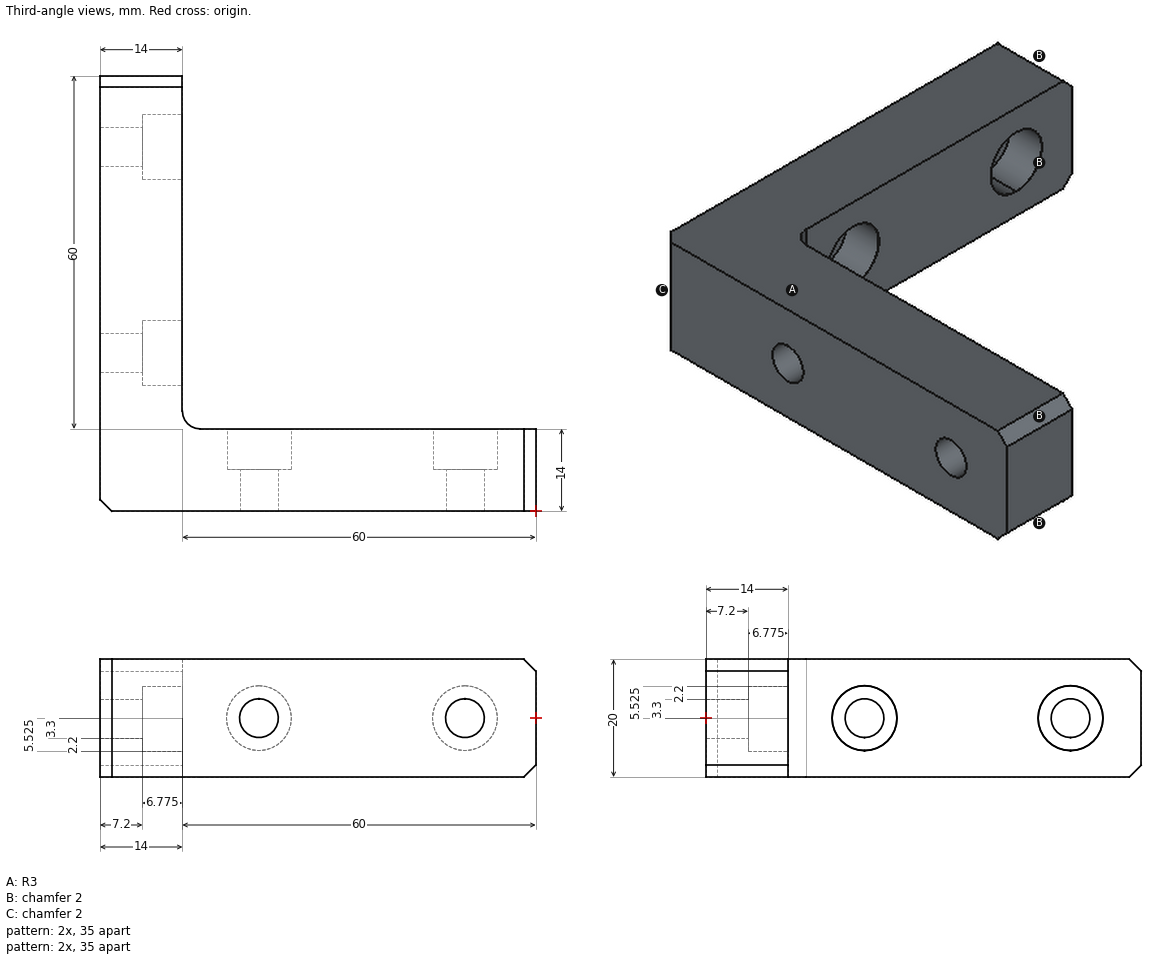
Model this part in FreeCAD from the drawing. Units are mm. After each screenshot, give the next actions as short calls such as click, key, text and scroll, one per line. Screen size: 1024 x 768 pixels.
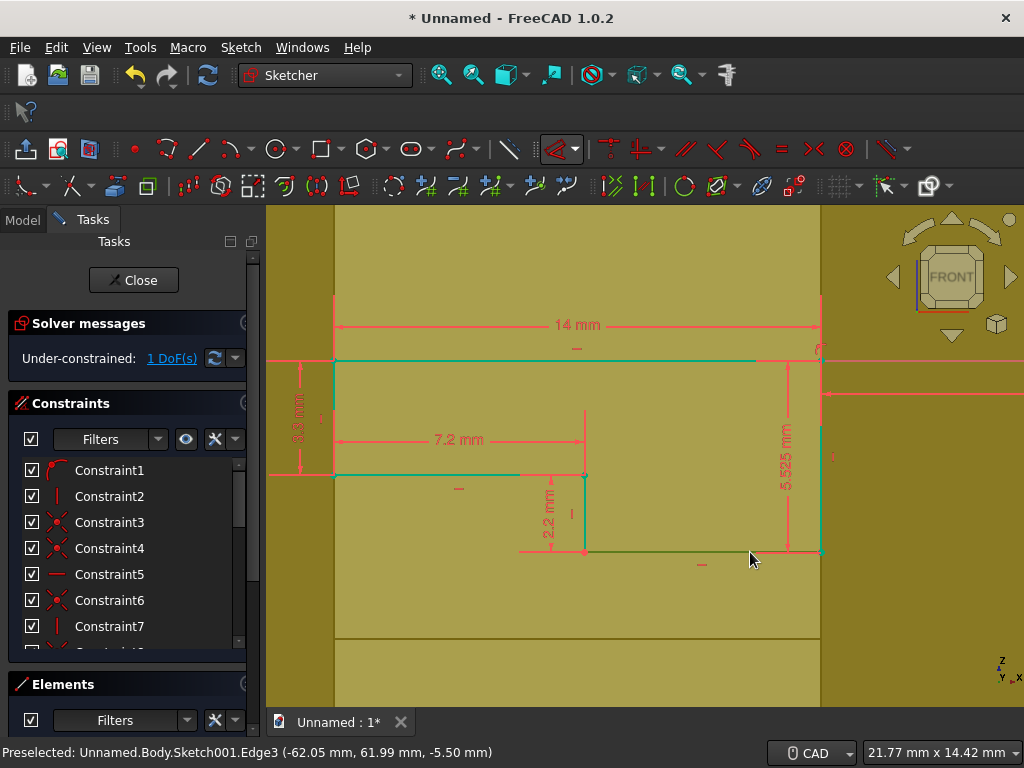
click(578, 150)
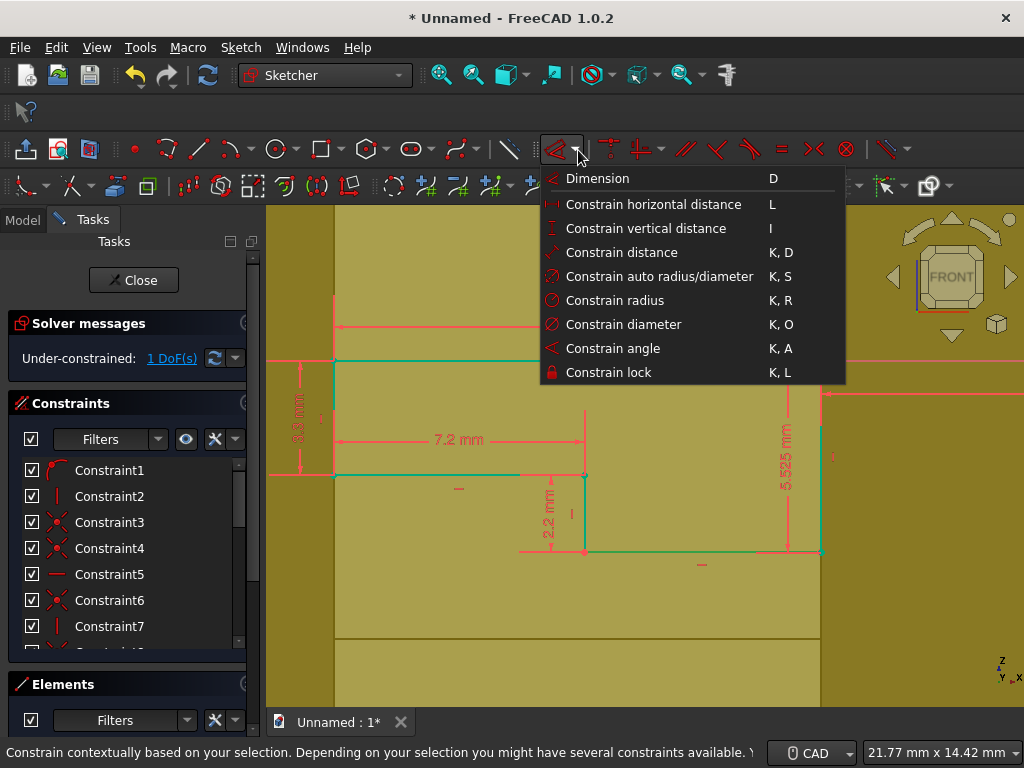
click(693, 204)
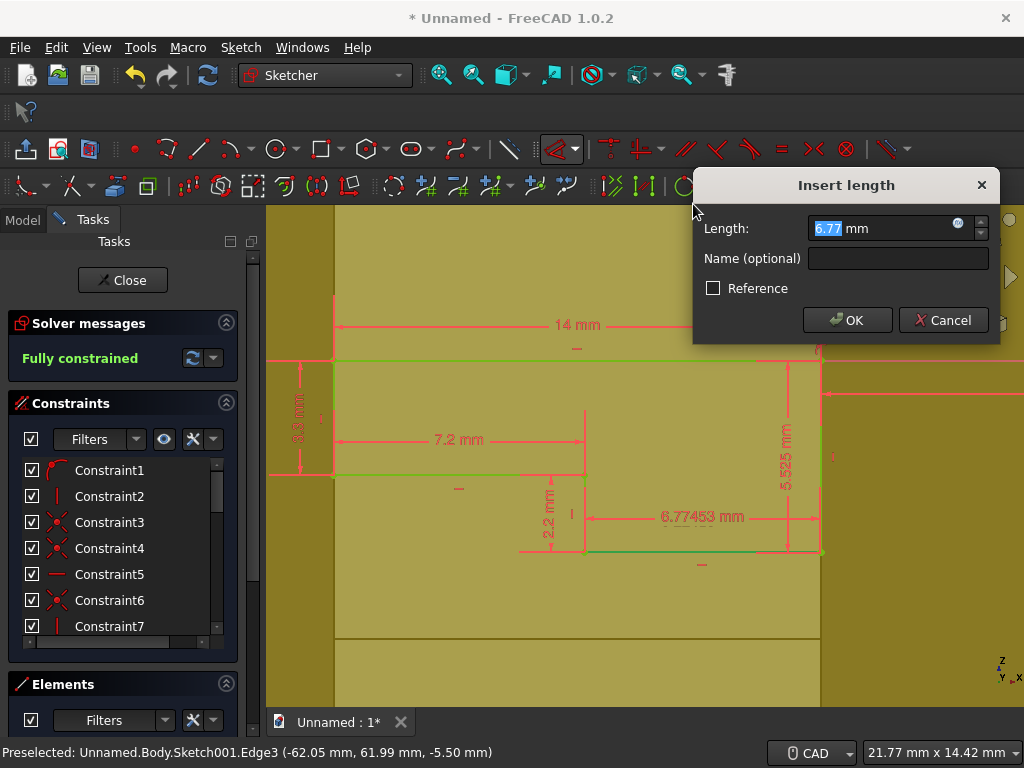
text(6.775)
key(Return)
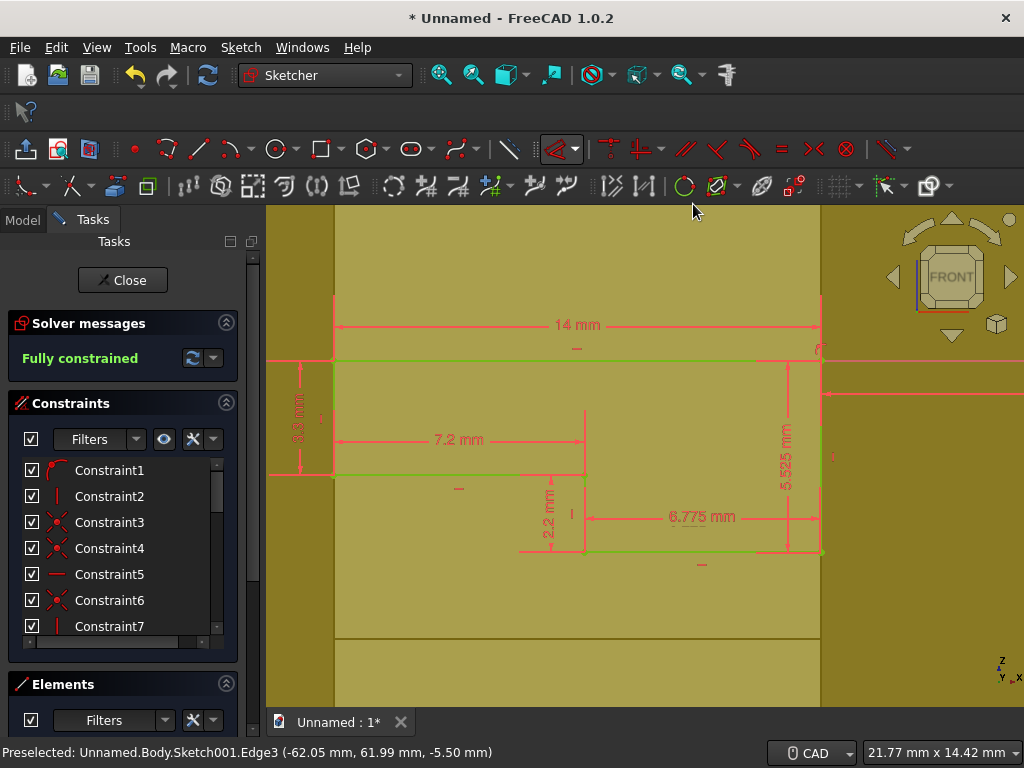
click(123, 280)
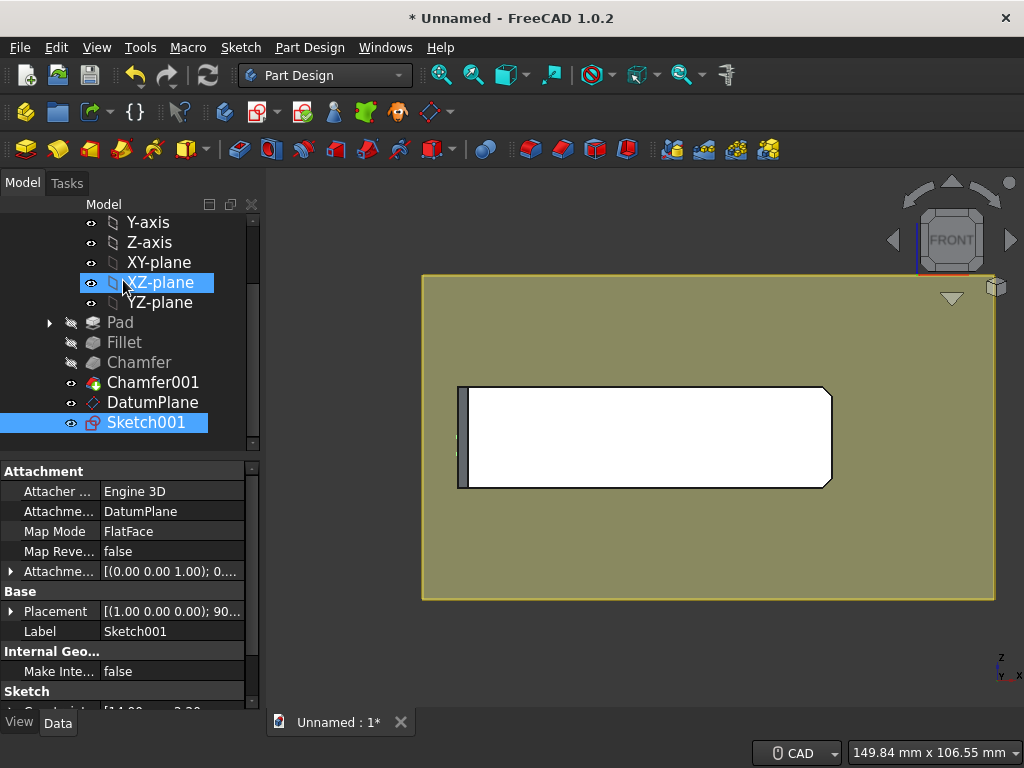
click(304, 150)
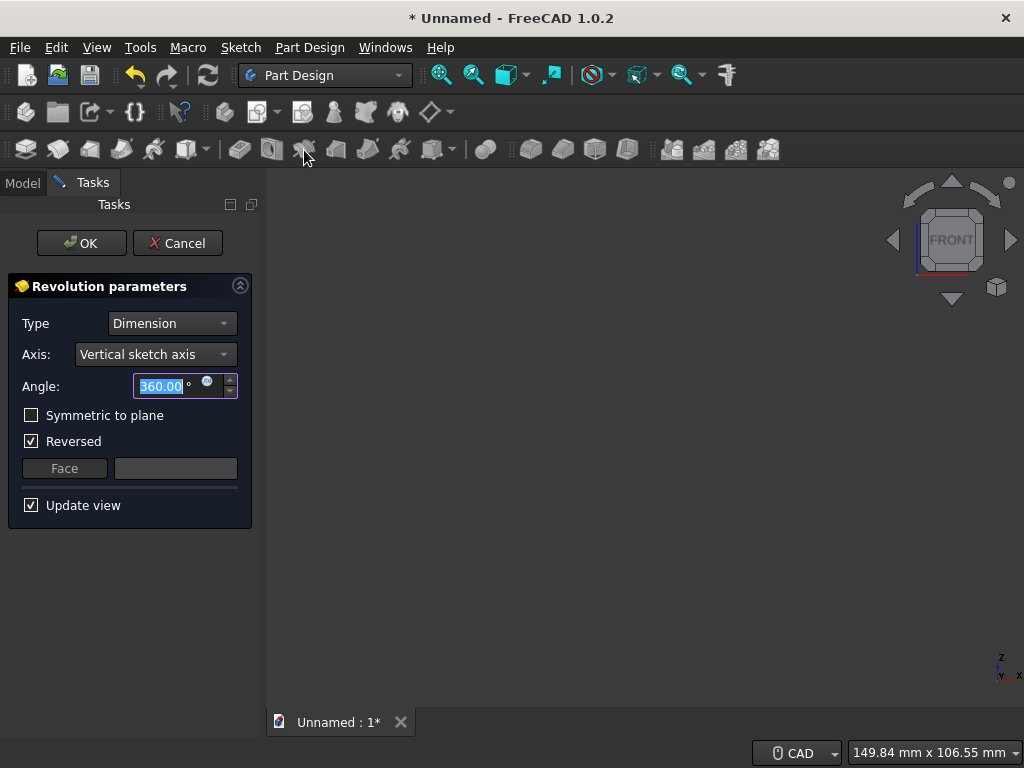
click(156, 354)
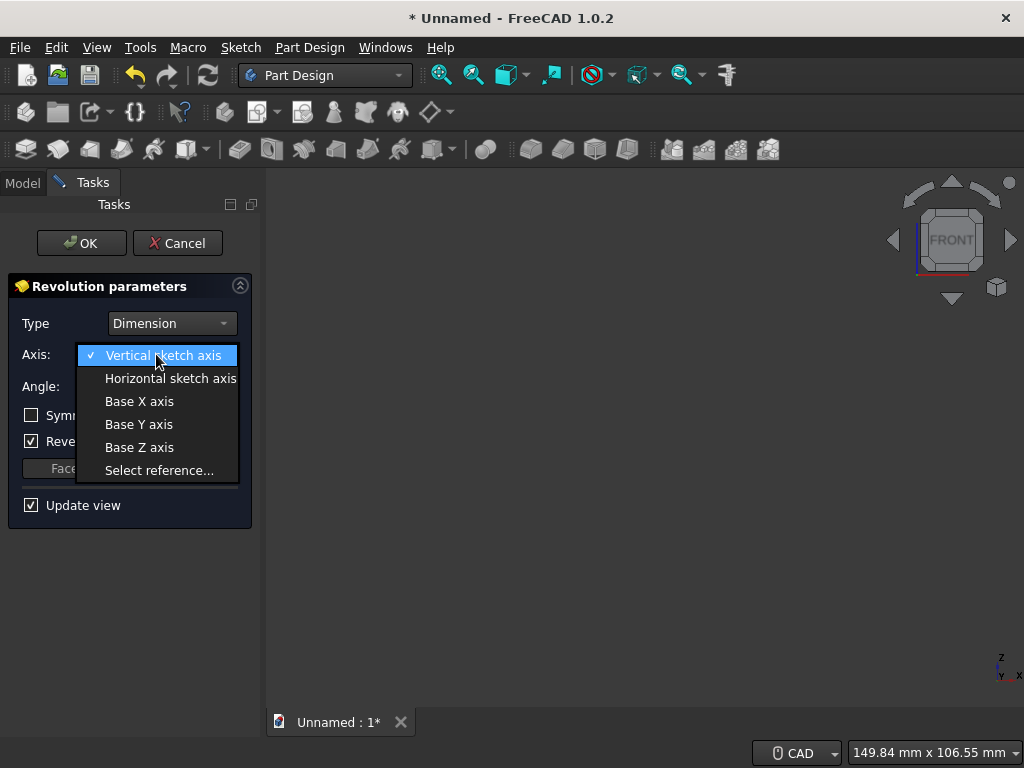
click(156, 378)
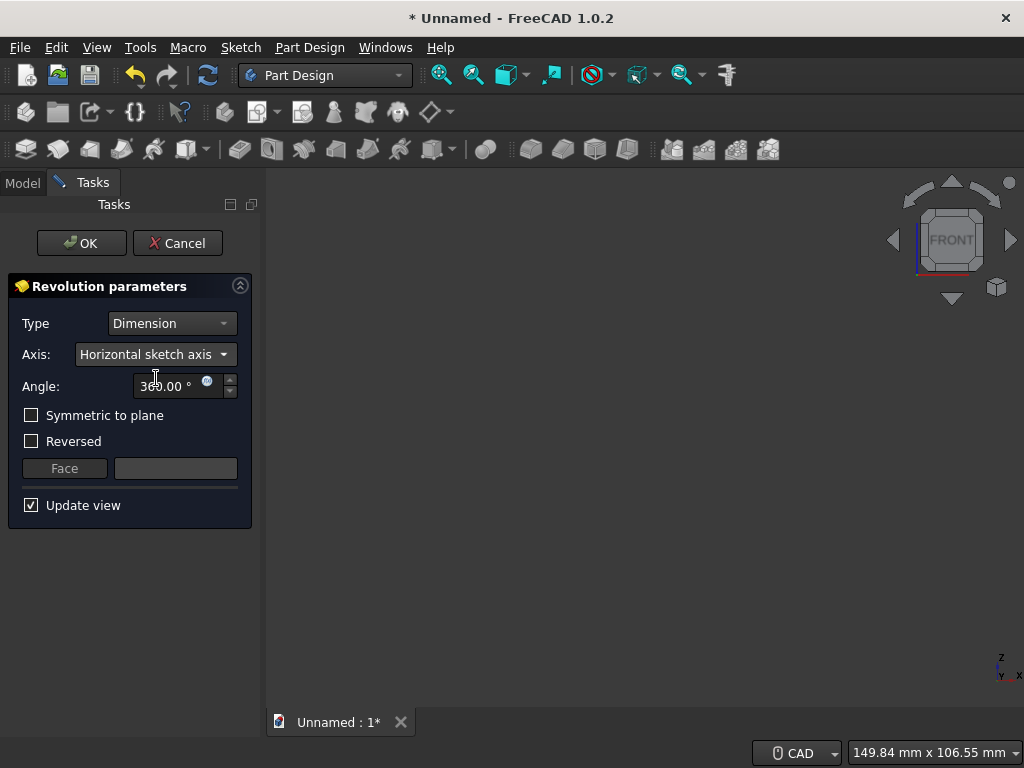
click(82, 243)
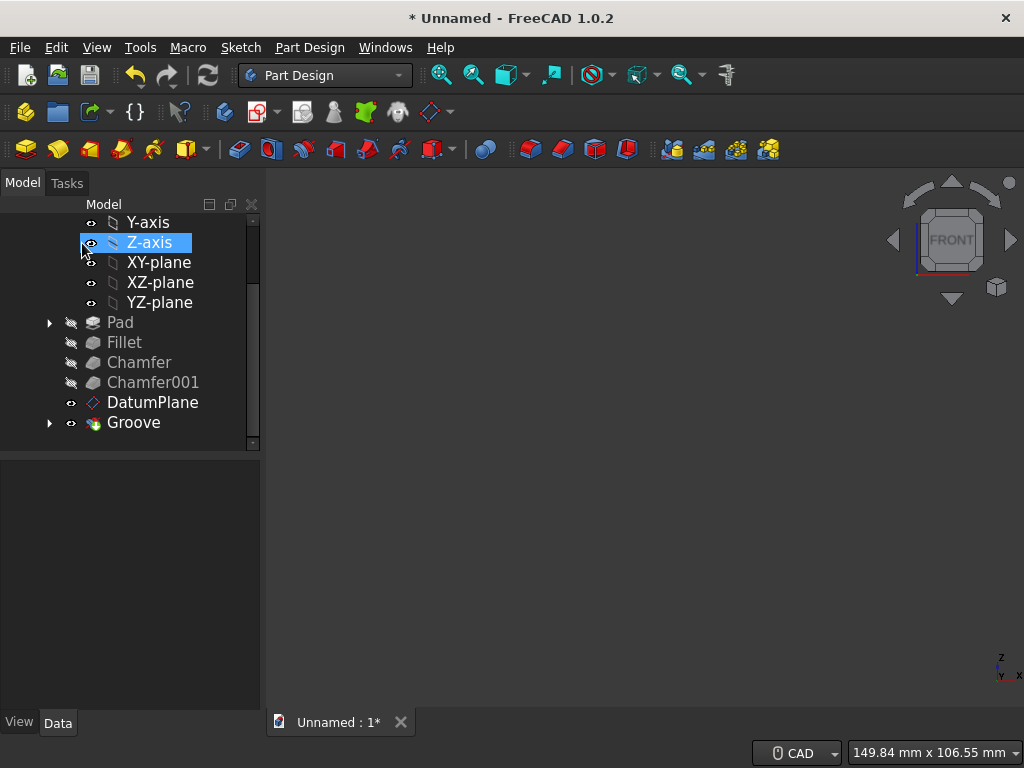
click(116, 403)
key(space)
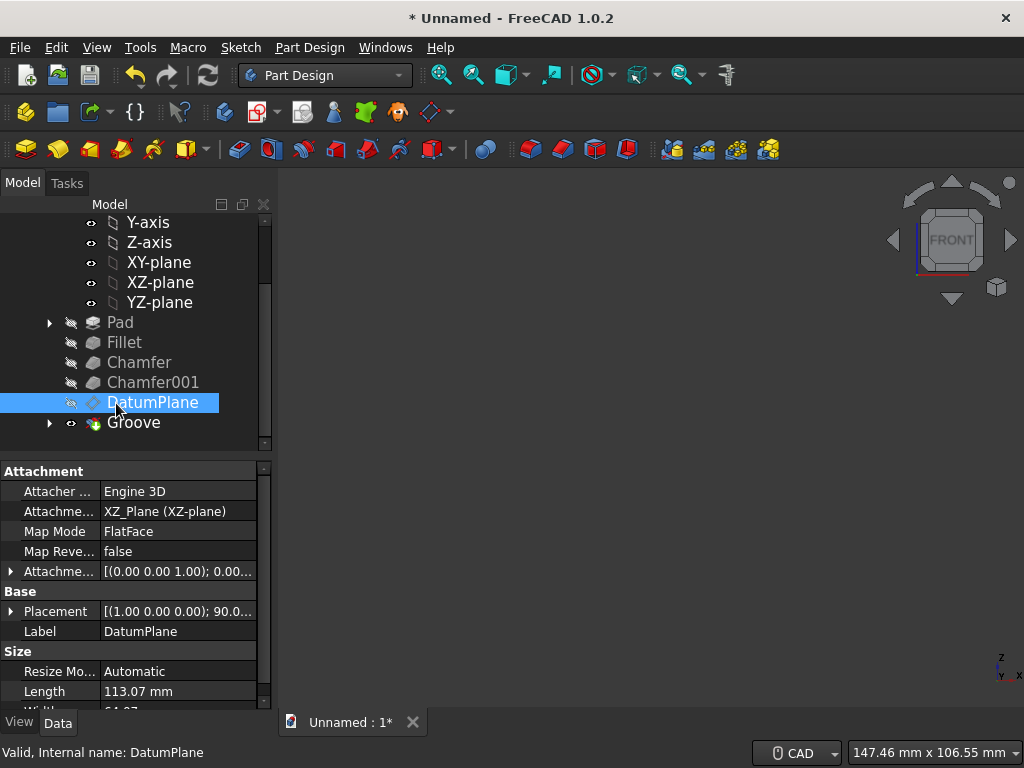
click(442, 76)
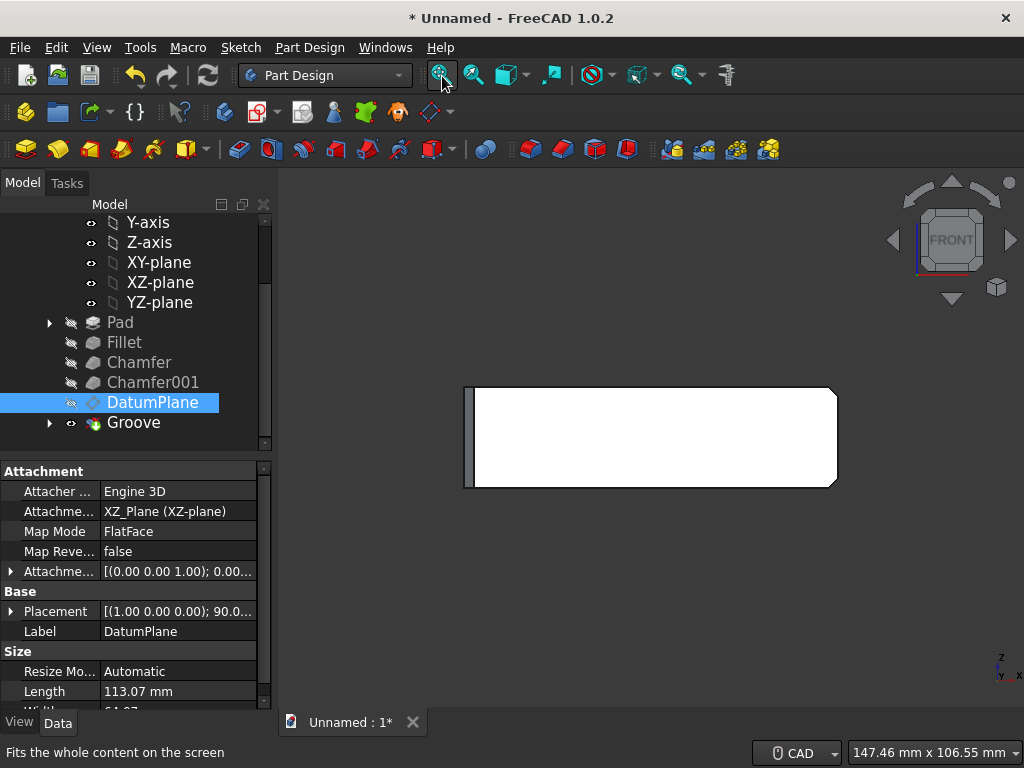
click(116, 423)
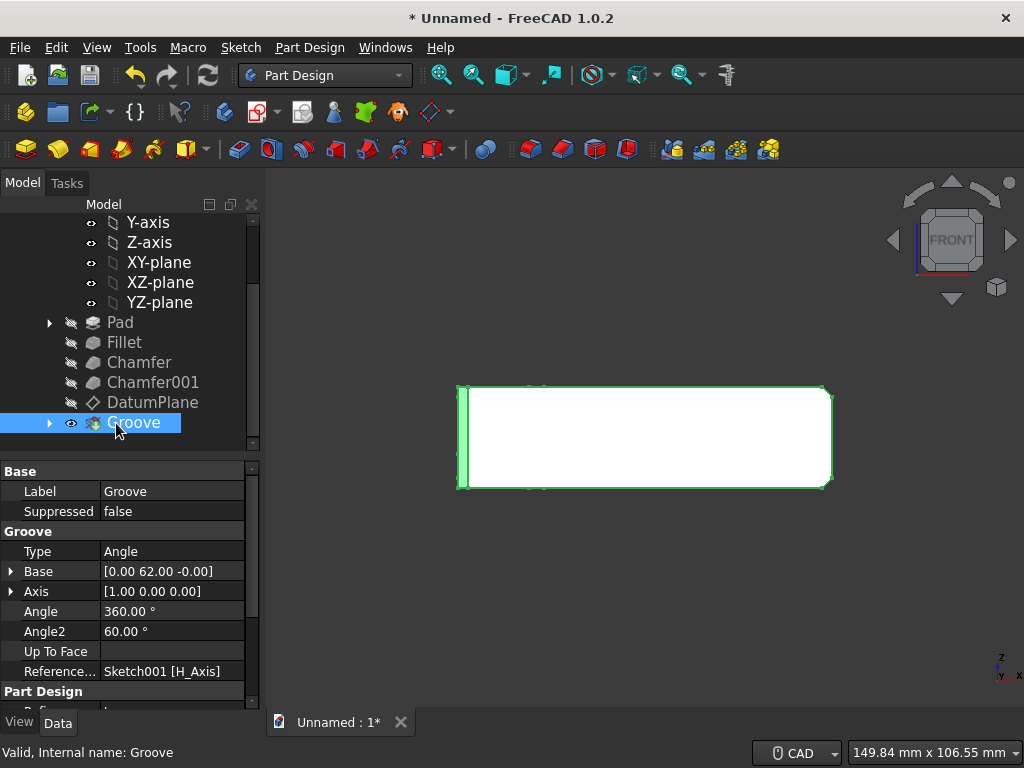
click(704, 150)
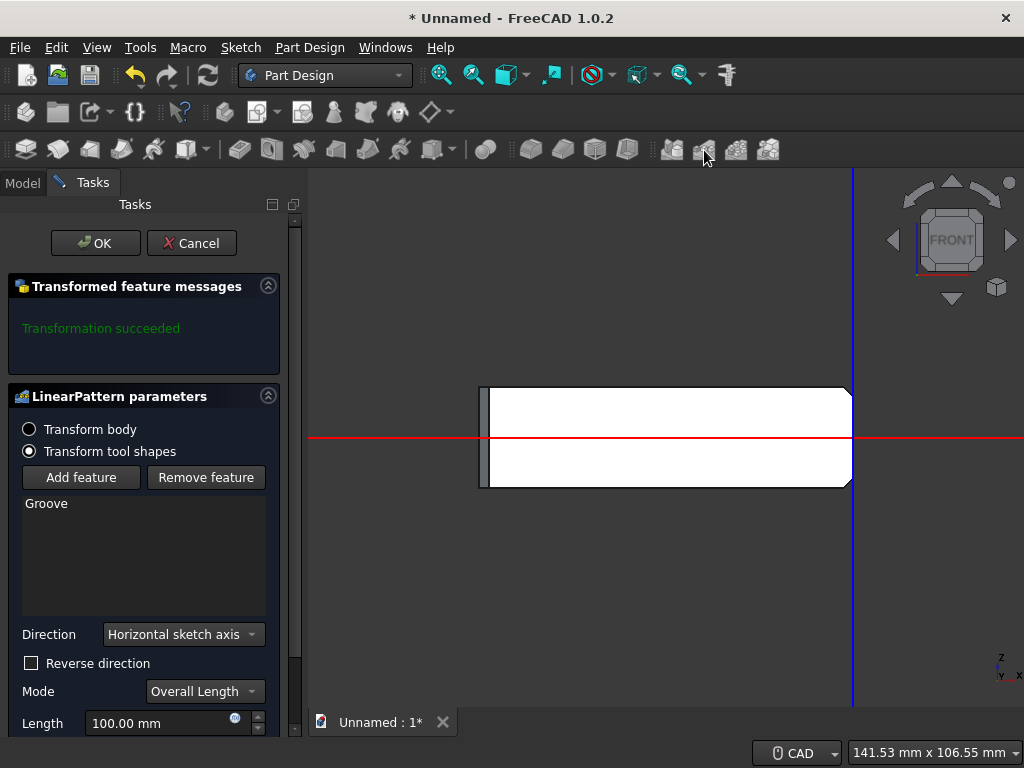
click(184, 634)